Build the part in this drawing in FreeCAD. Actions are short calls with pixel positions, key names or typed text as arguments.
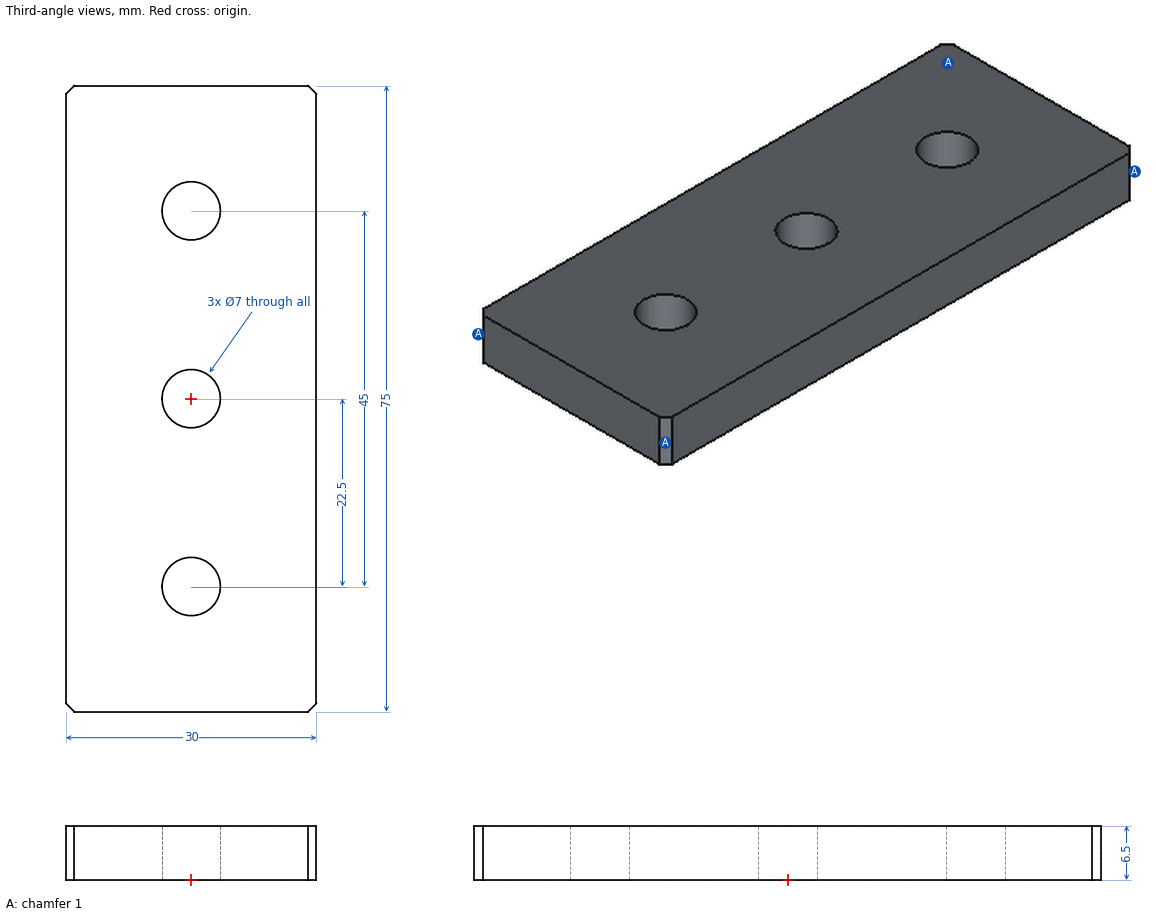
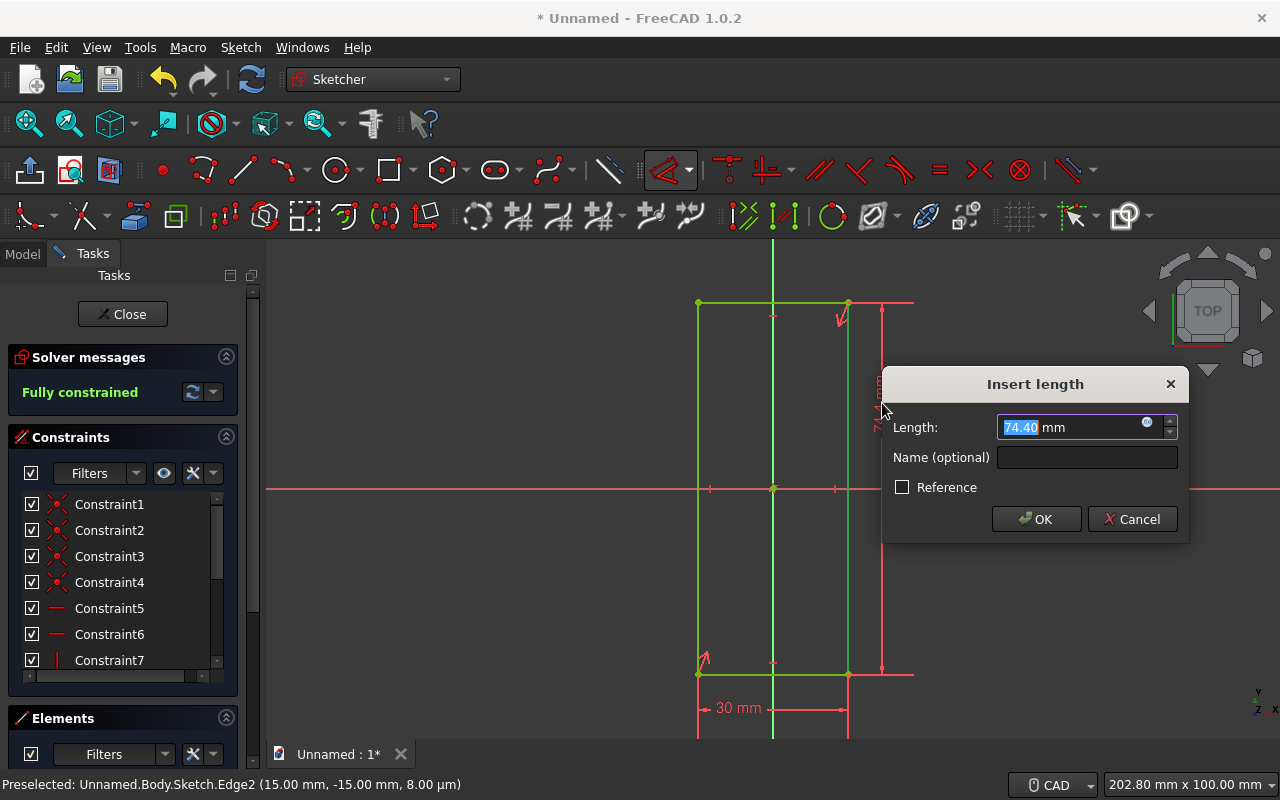
text(75)
key(Return)
key(Escape)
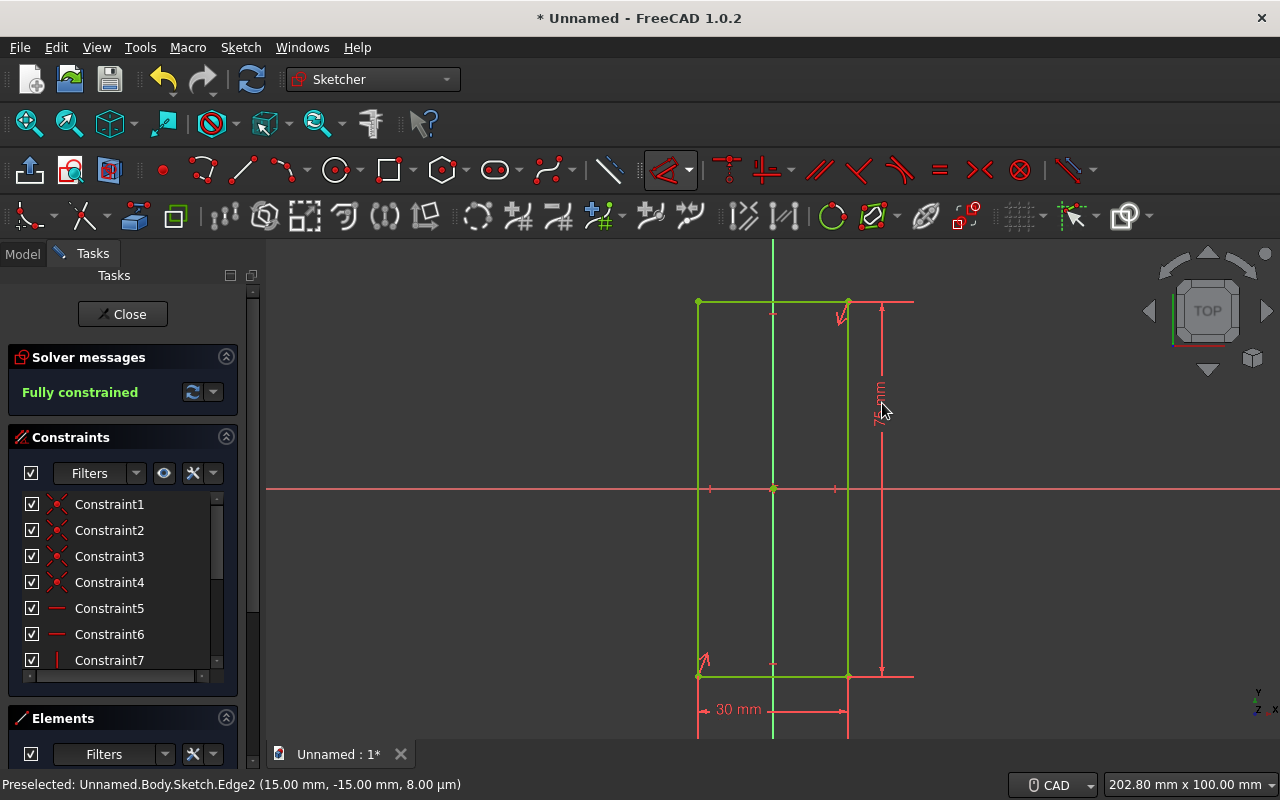
click(123, 314)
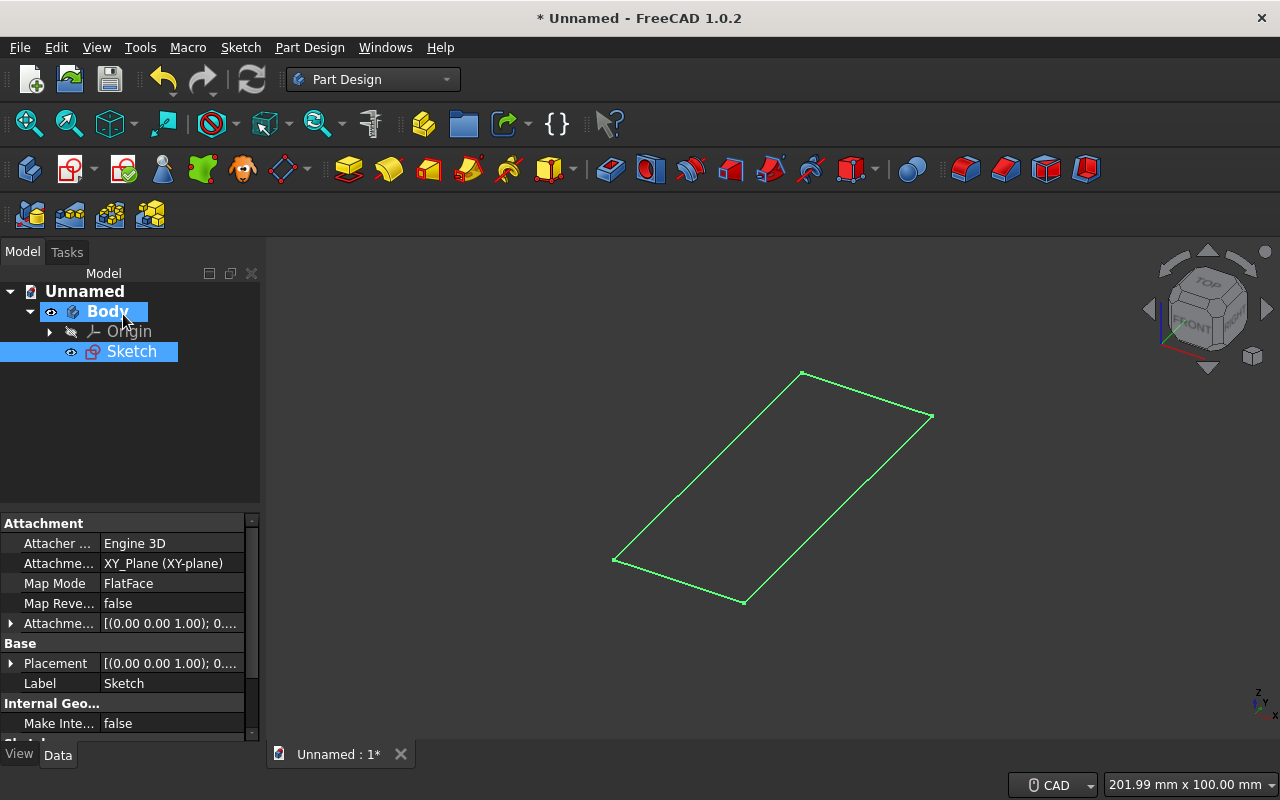
click(350, 170)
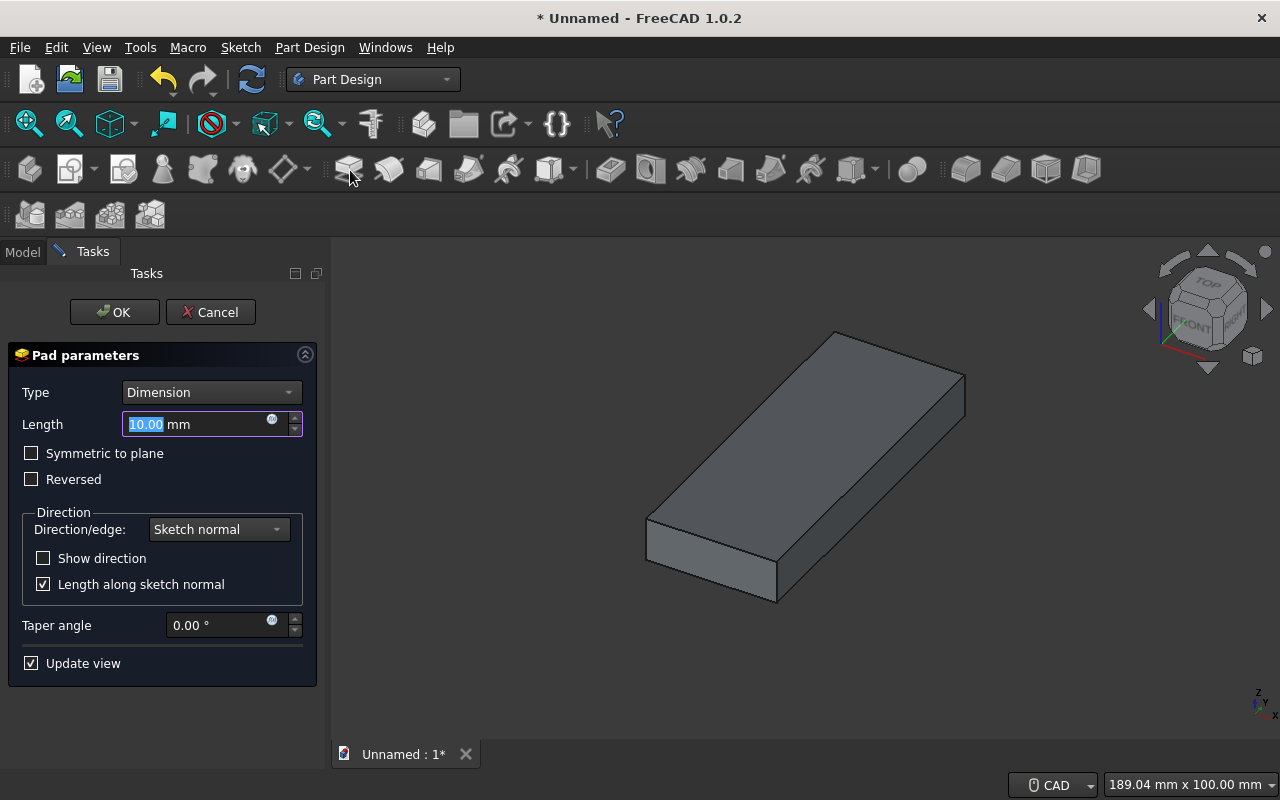
text(6.5)
key(Tab)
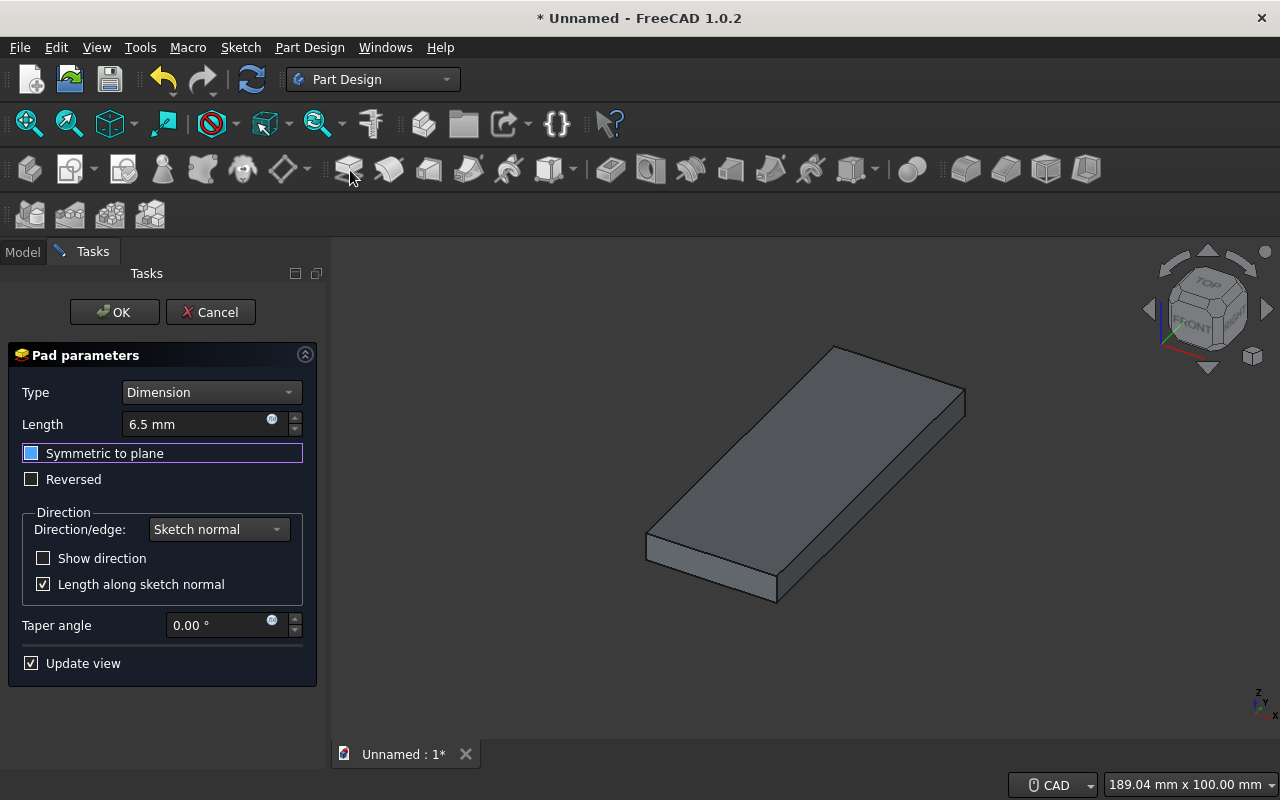
click(115, 312)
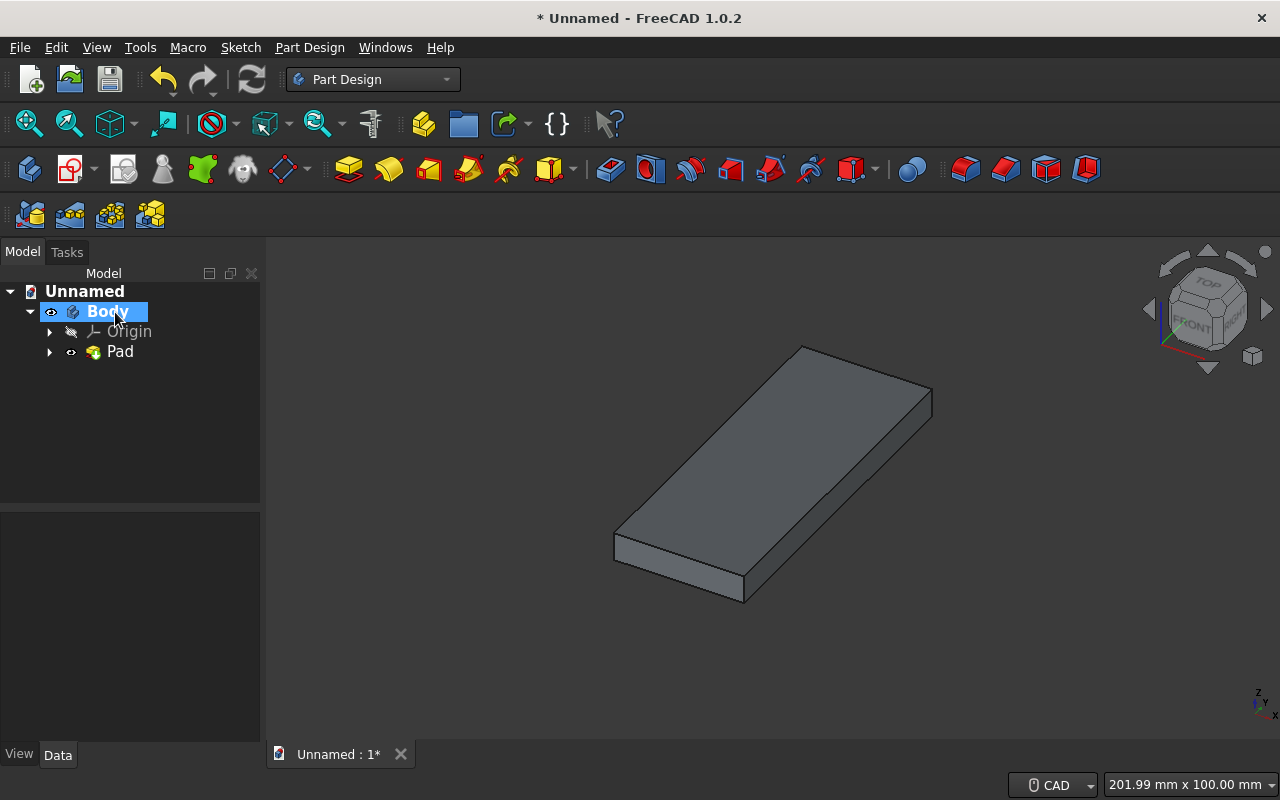
click(827, 407)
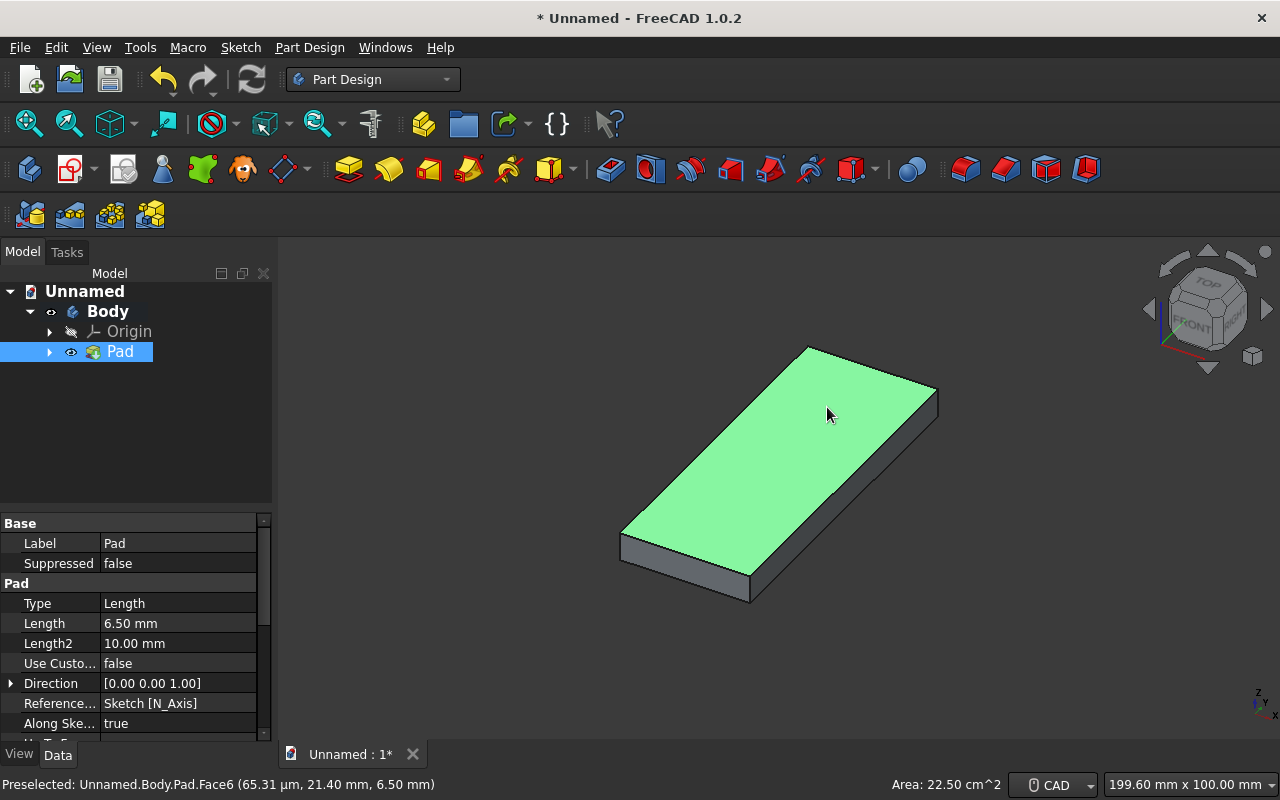
click(70, 170)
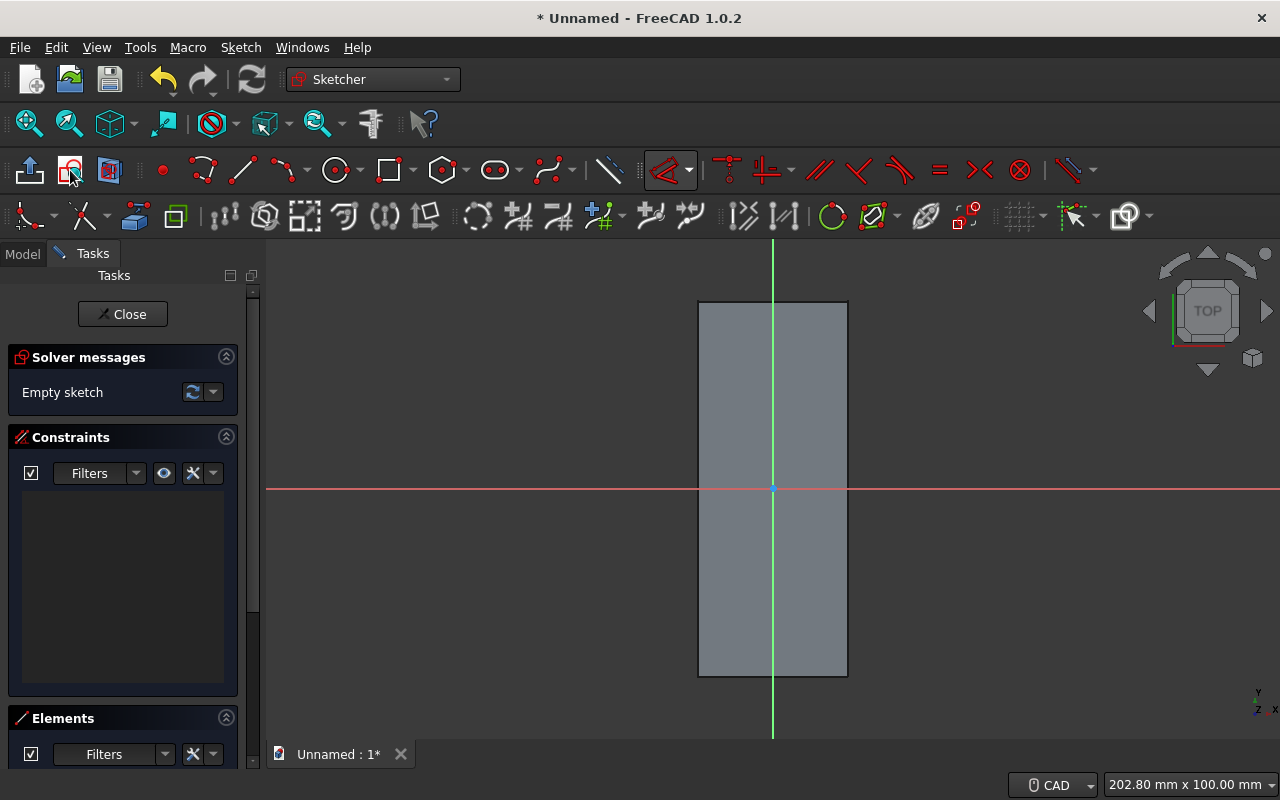
click(336, 170)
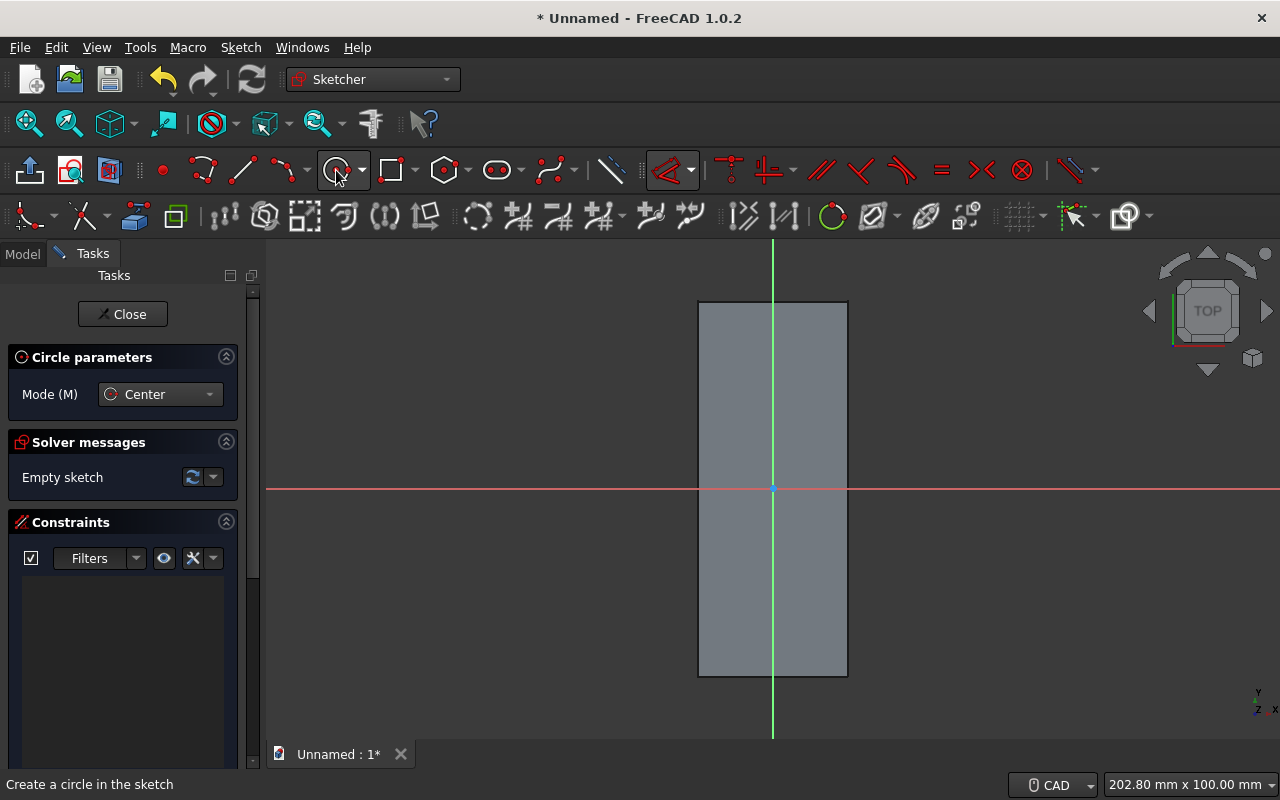
scroll(773, 489, up, 2)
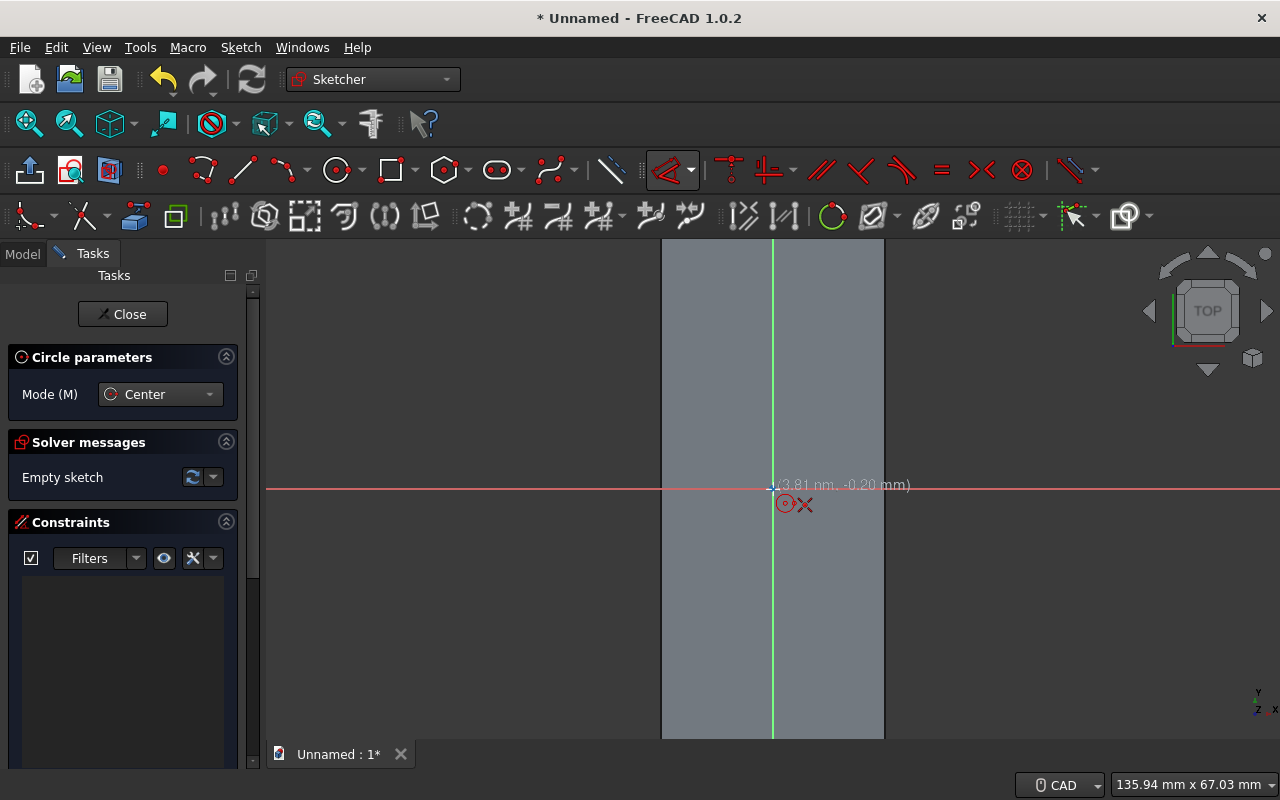
click(773, 489)
click(791, 470)